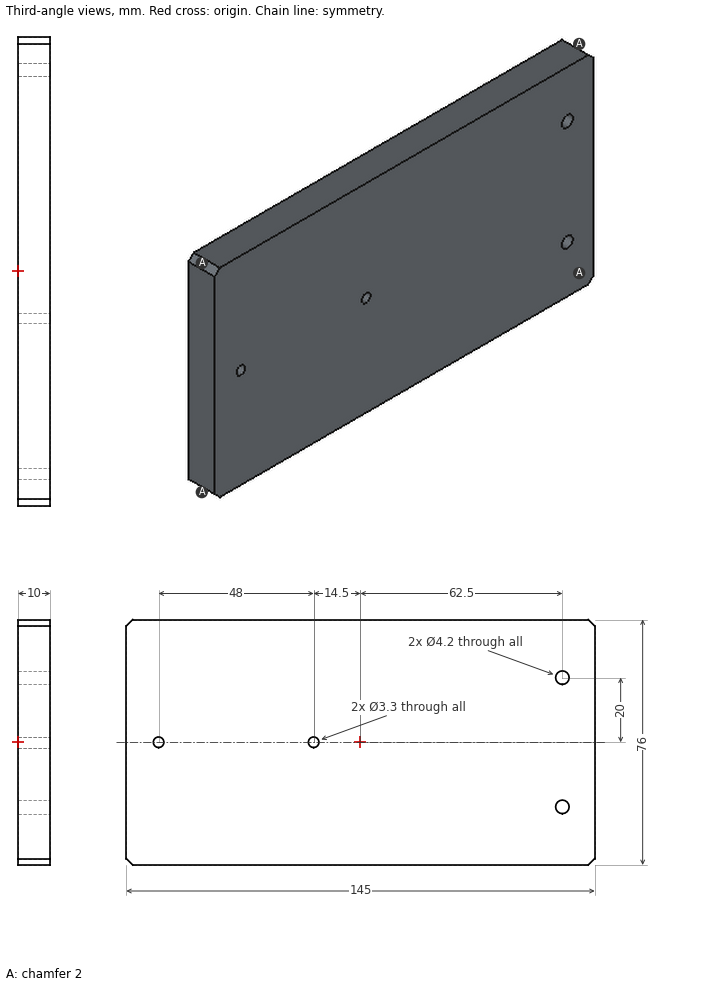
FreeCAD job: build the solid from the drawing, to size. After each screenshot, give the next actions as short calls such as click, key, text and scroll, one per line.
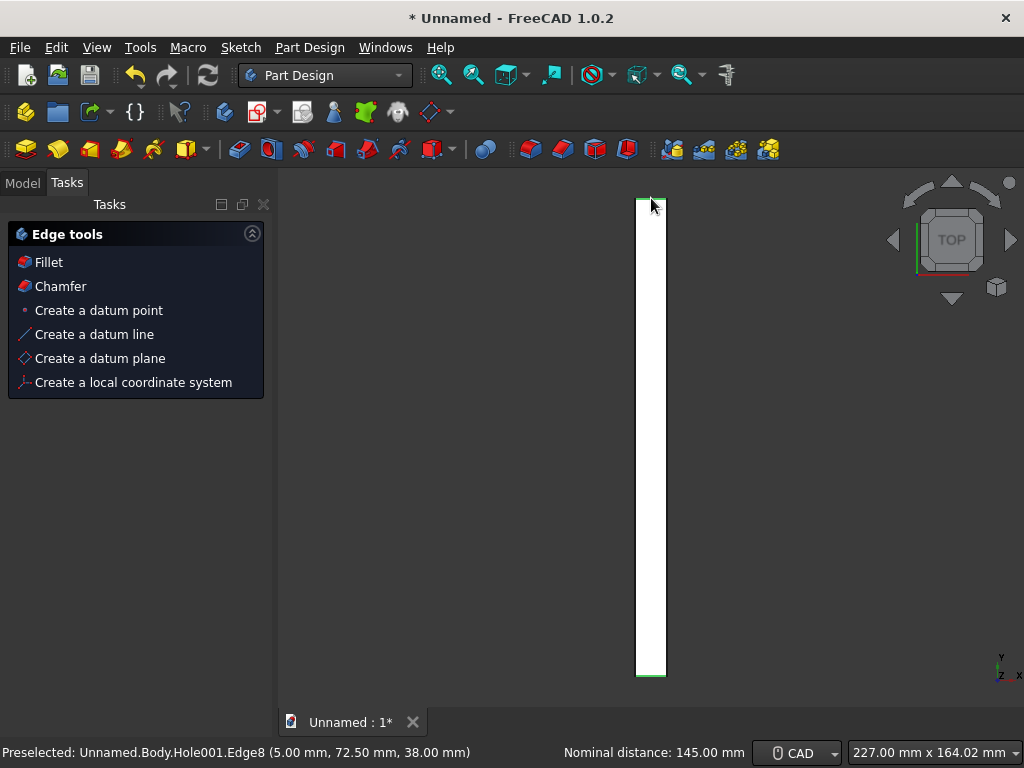
key(1)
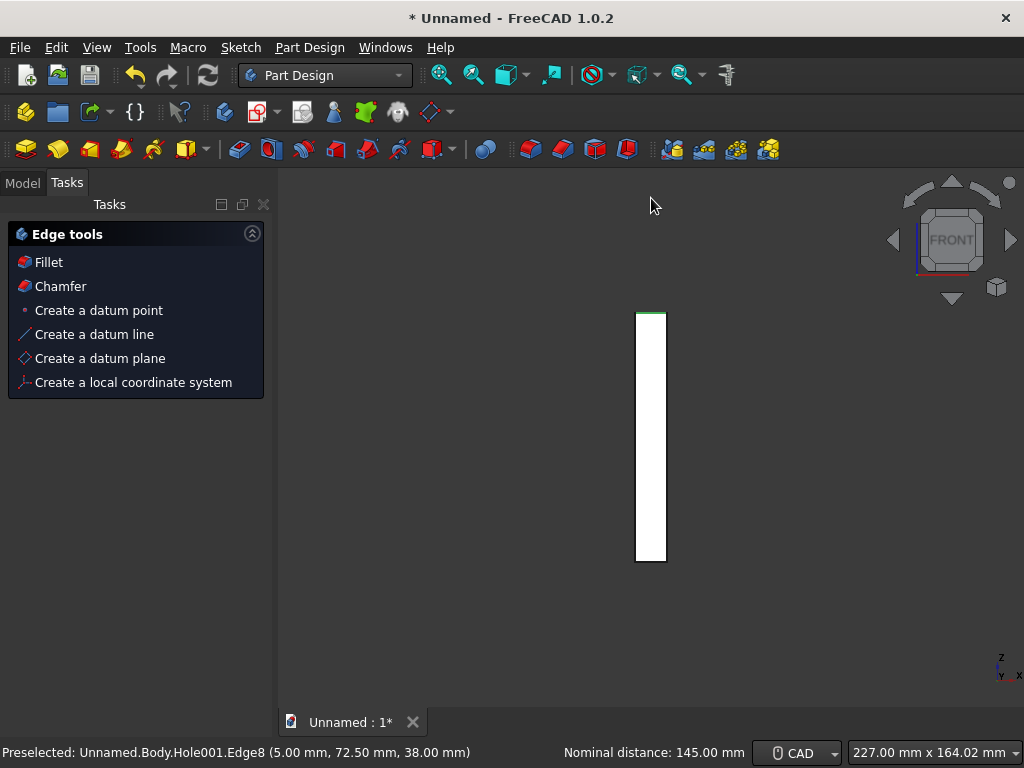
click(651, 561, ctrl)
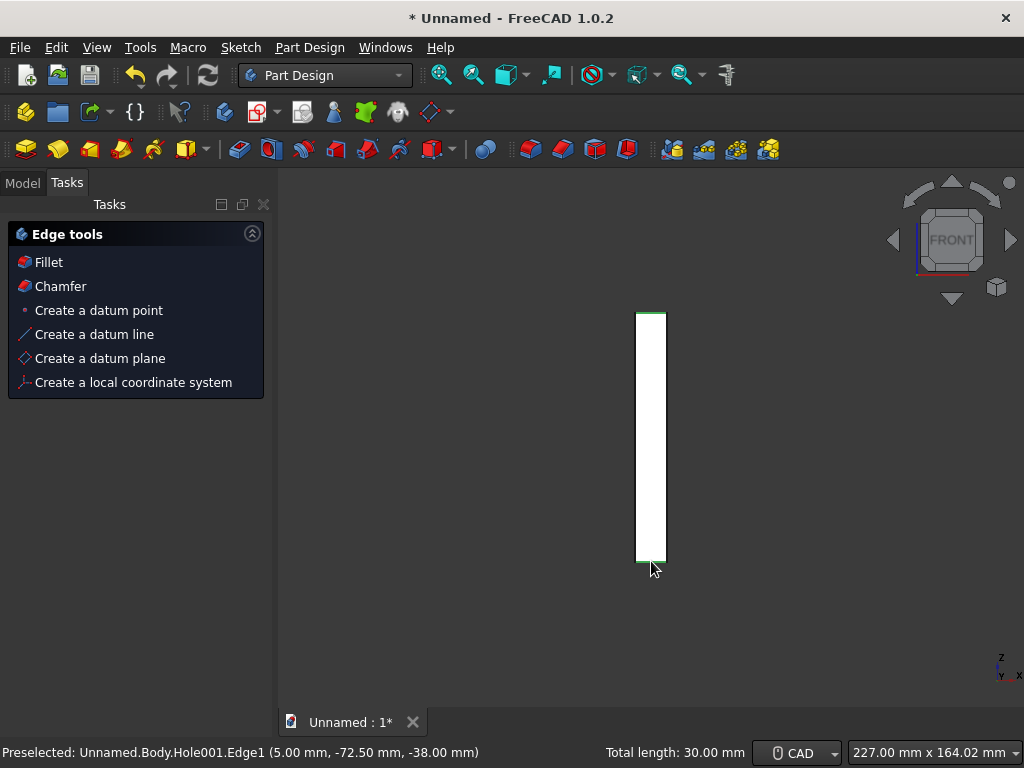
key(3)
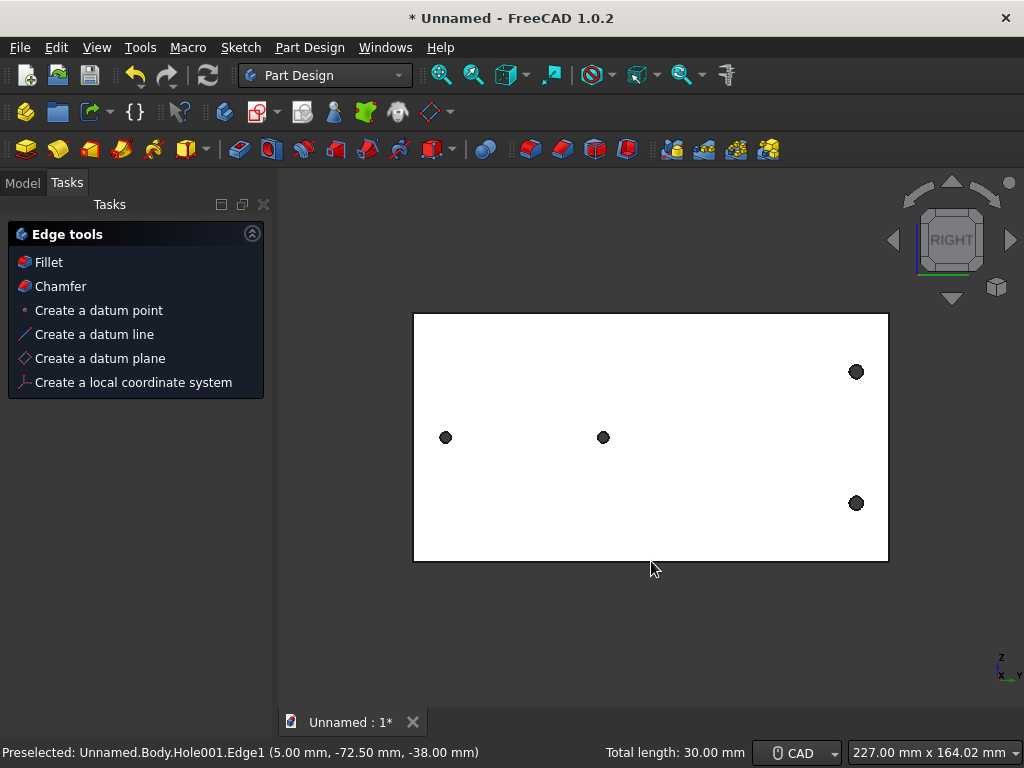
key(5)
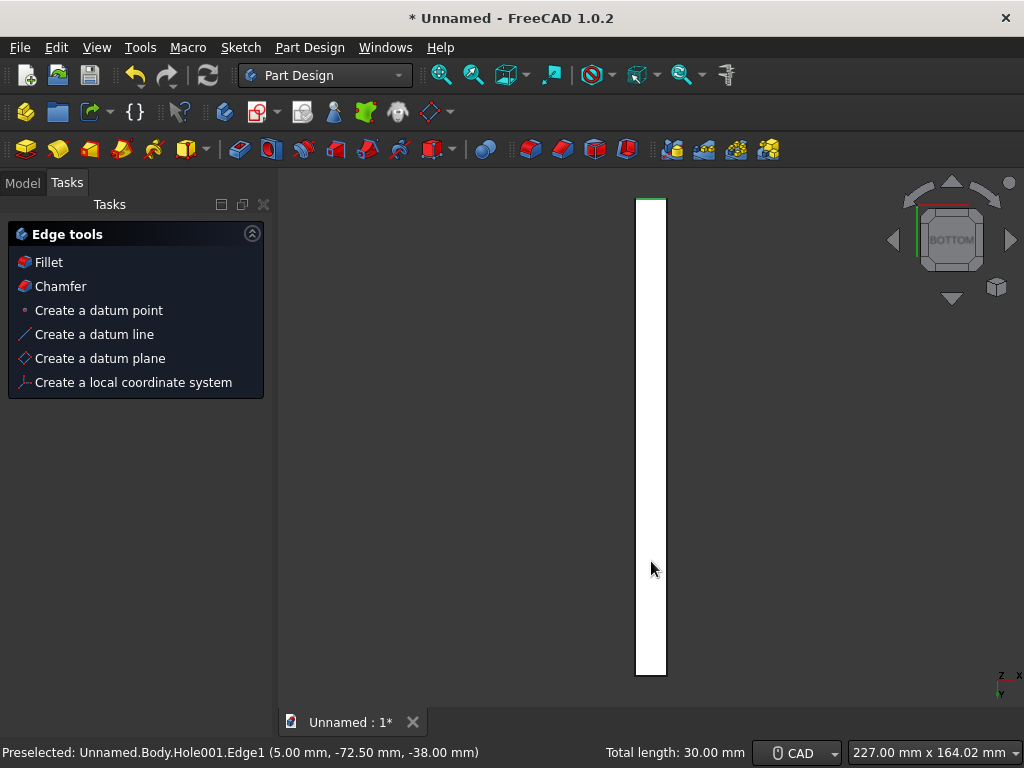
click(651, 675, ctrl)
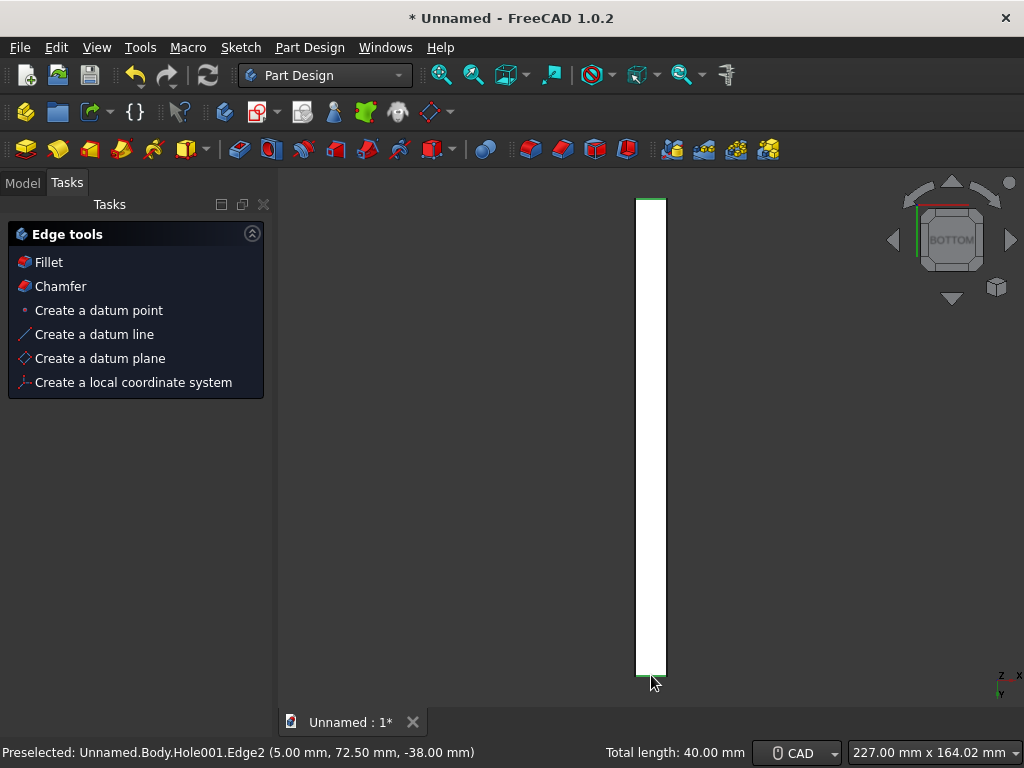
click(564, 150)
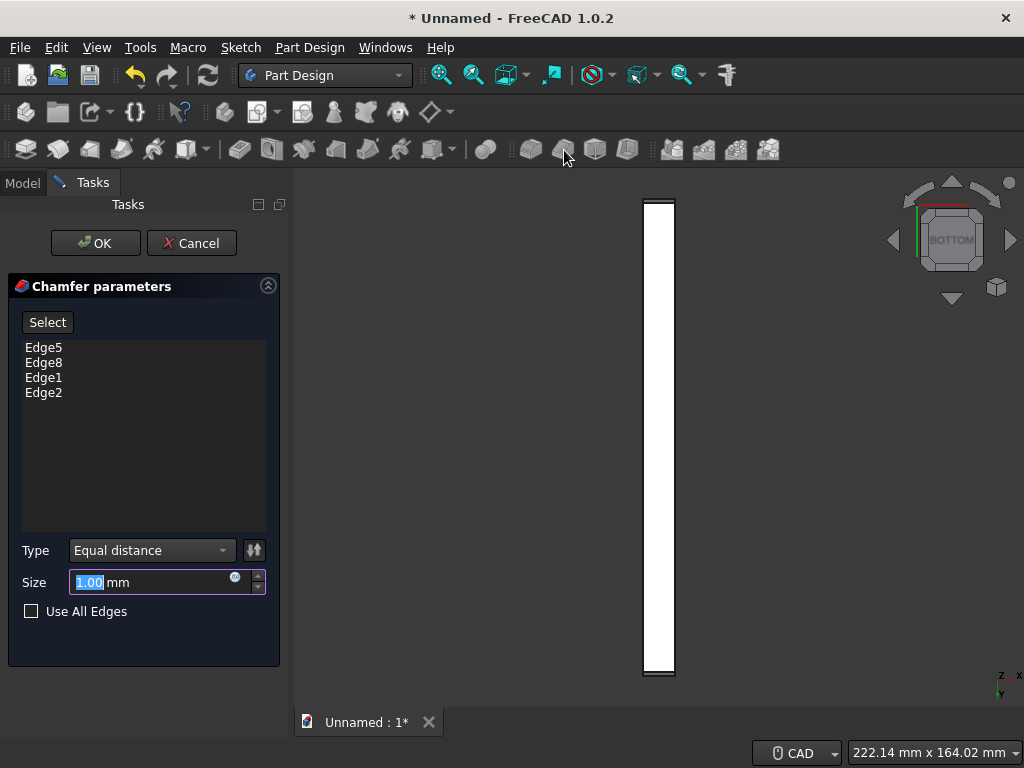
text(2)
key(Tab)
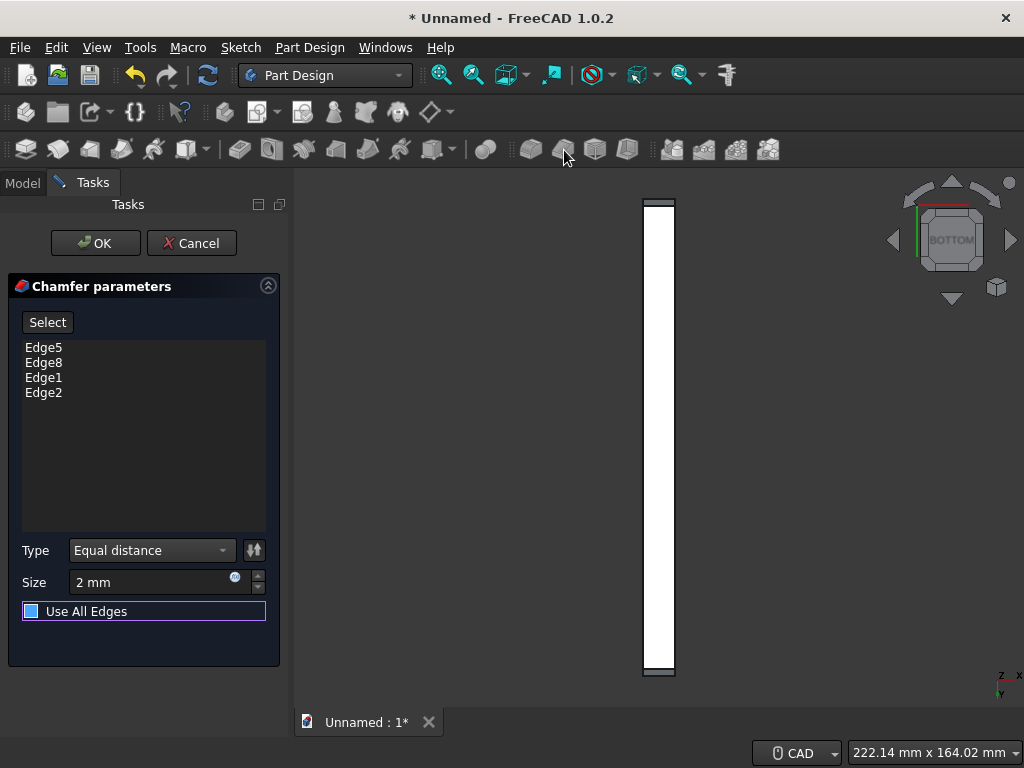
click(96, 243)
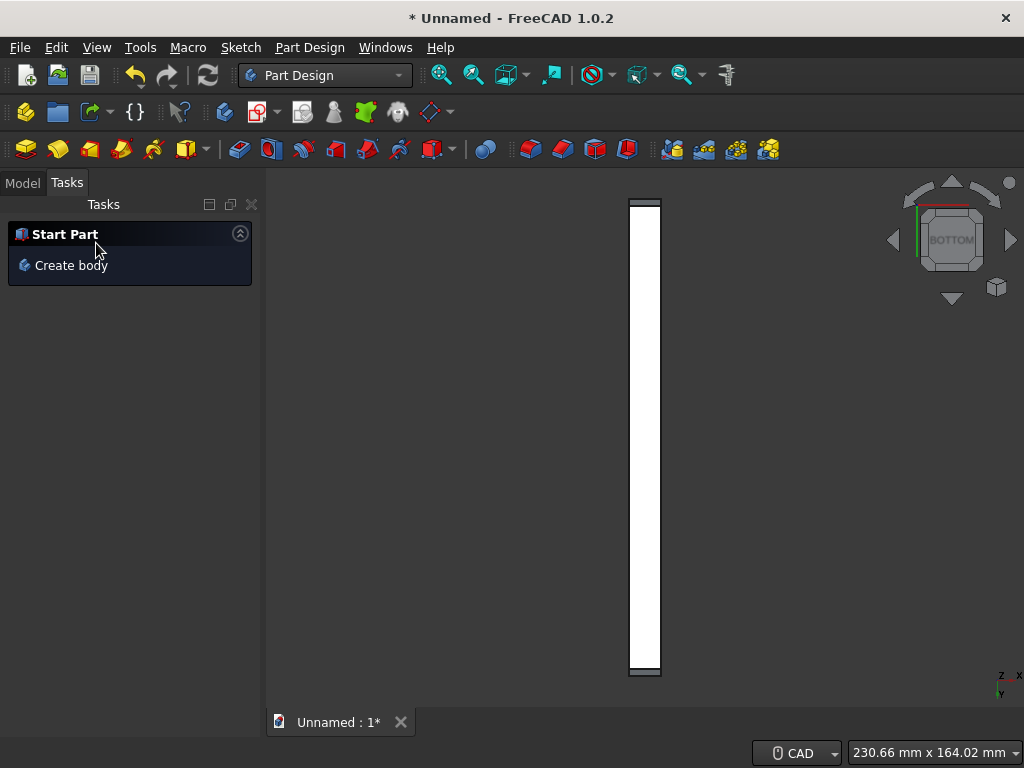
key(0)